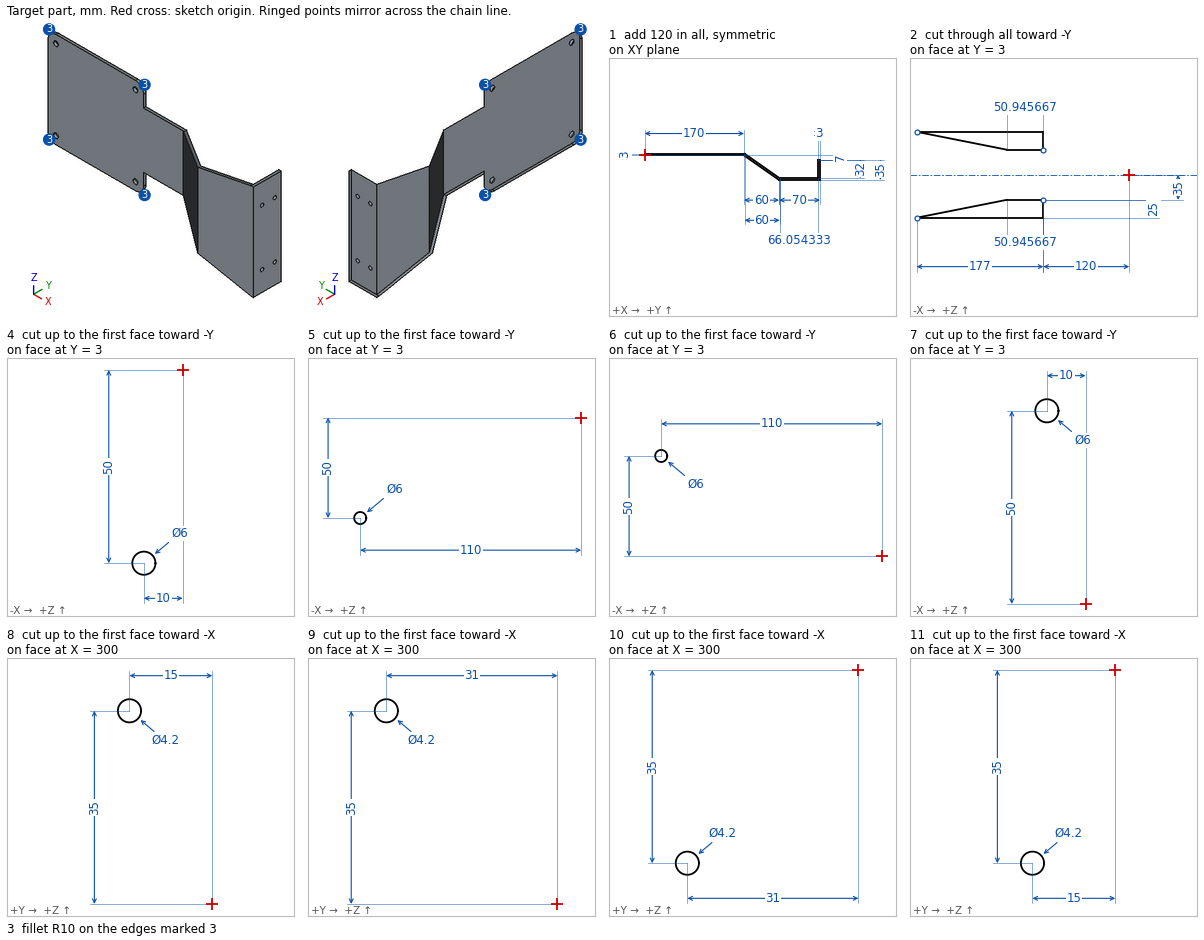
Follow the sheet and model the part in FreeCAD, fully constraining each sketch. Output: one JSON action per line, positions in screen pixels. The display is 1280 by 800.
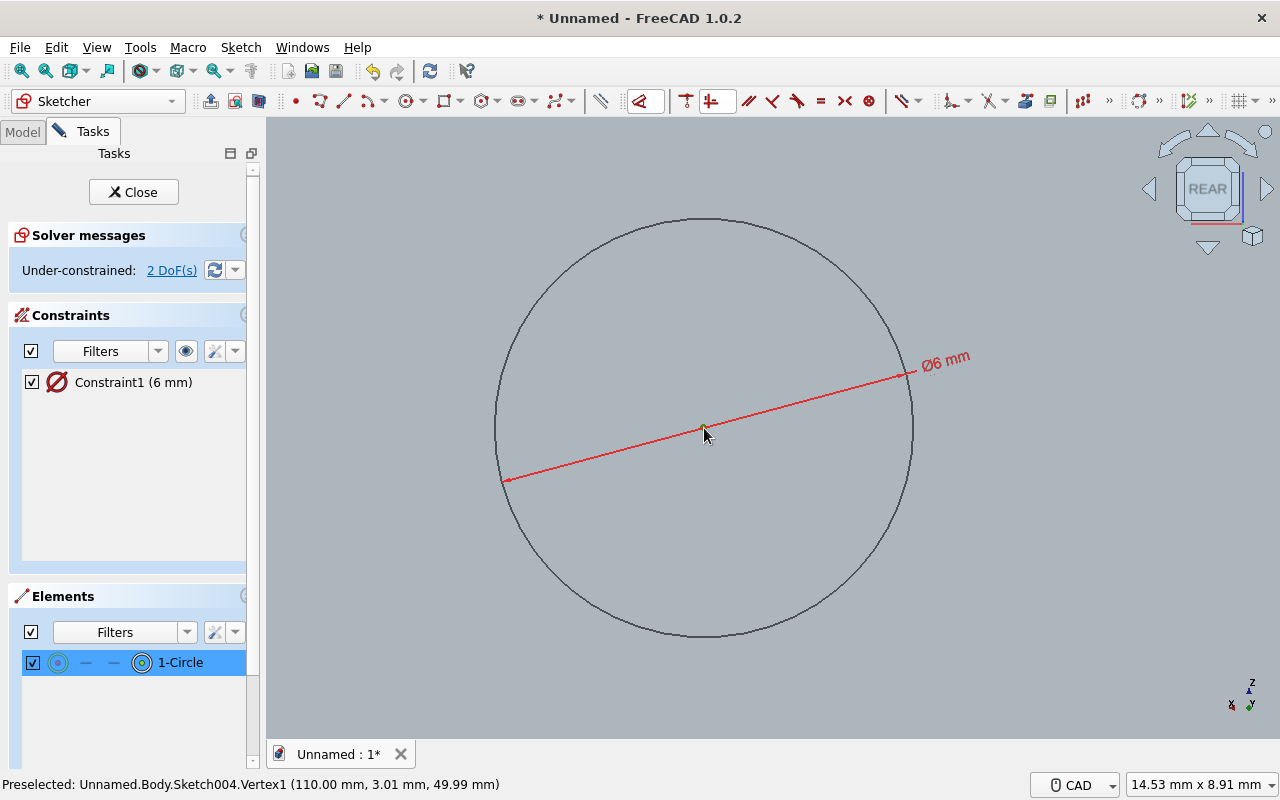
{"action": "left_click", "coordinate": [658, 102]}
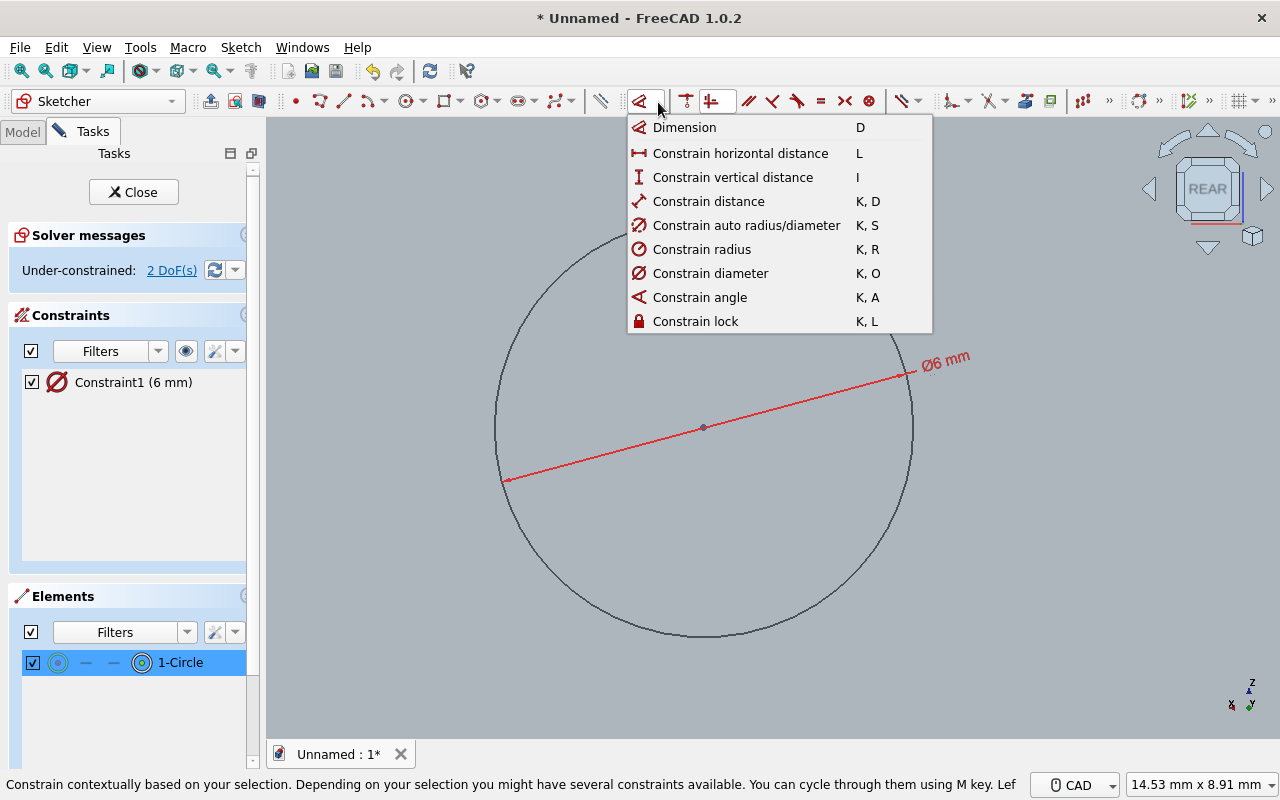
{"action": "left_click", "coordinate": [780, 177]}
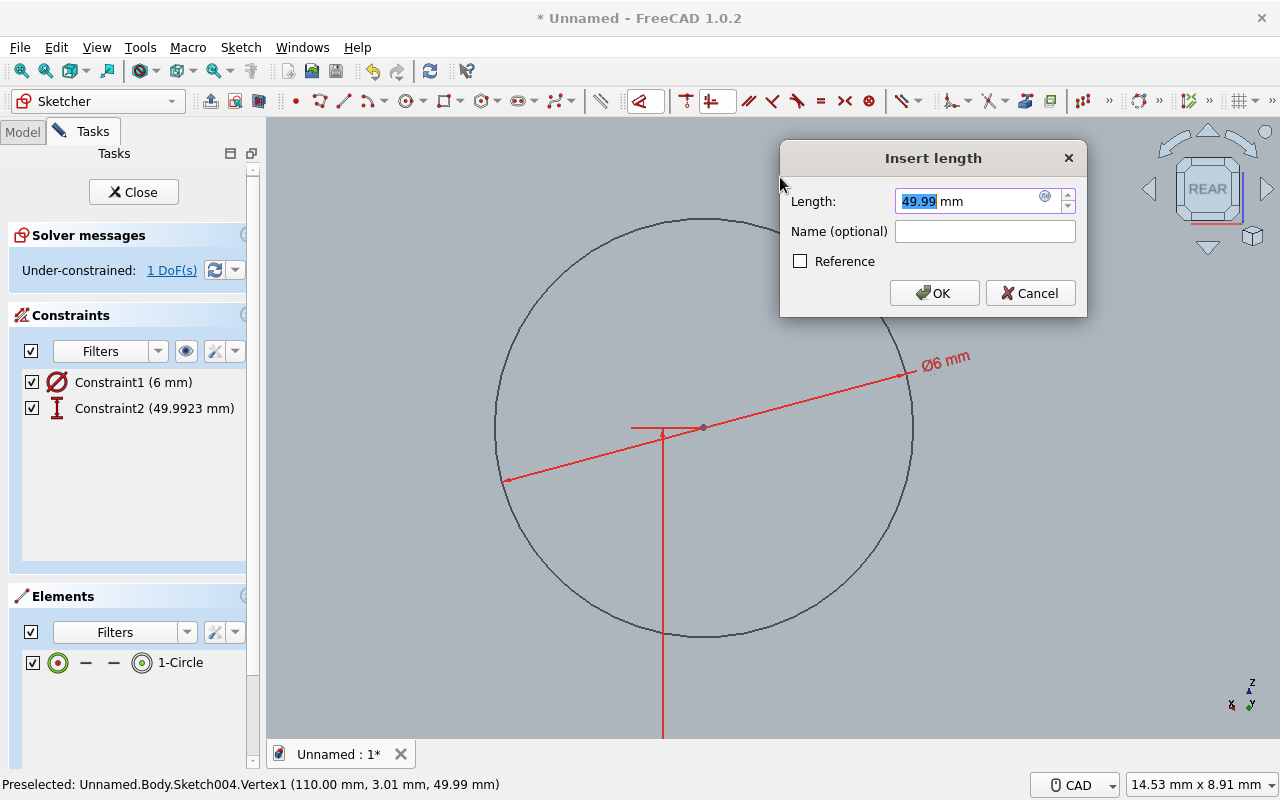
{"action": "type", "text": "50"}
{"action": "key", "text": "Return"}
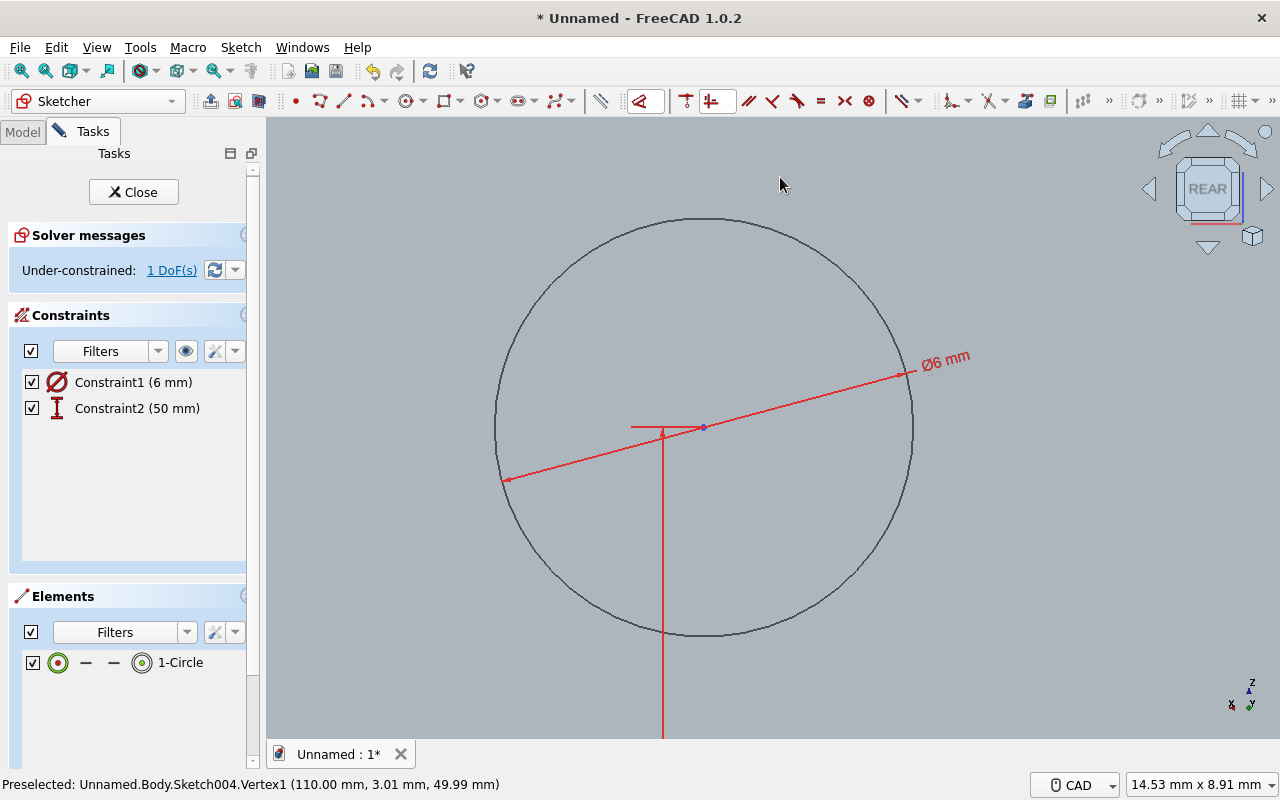
{"action": "left_click", "coordinate": [704, 427]}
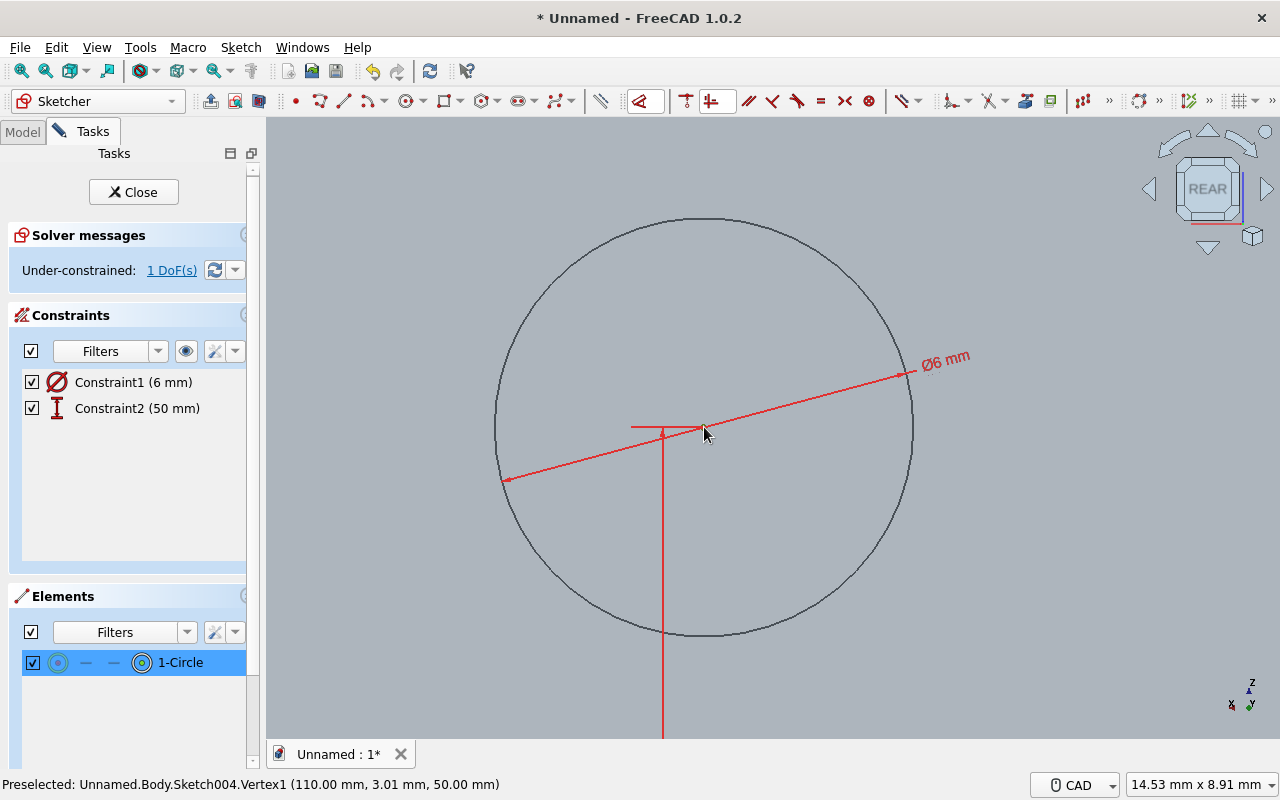
{"action": "left_click", "coordinate": [658, 102]}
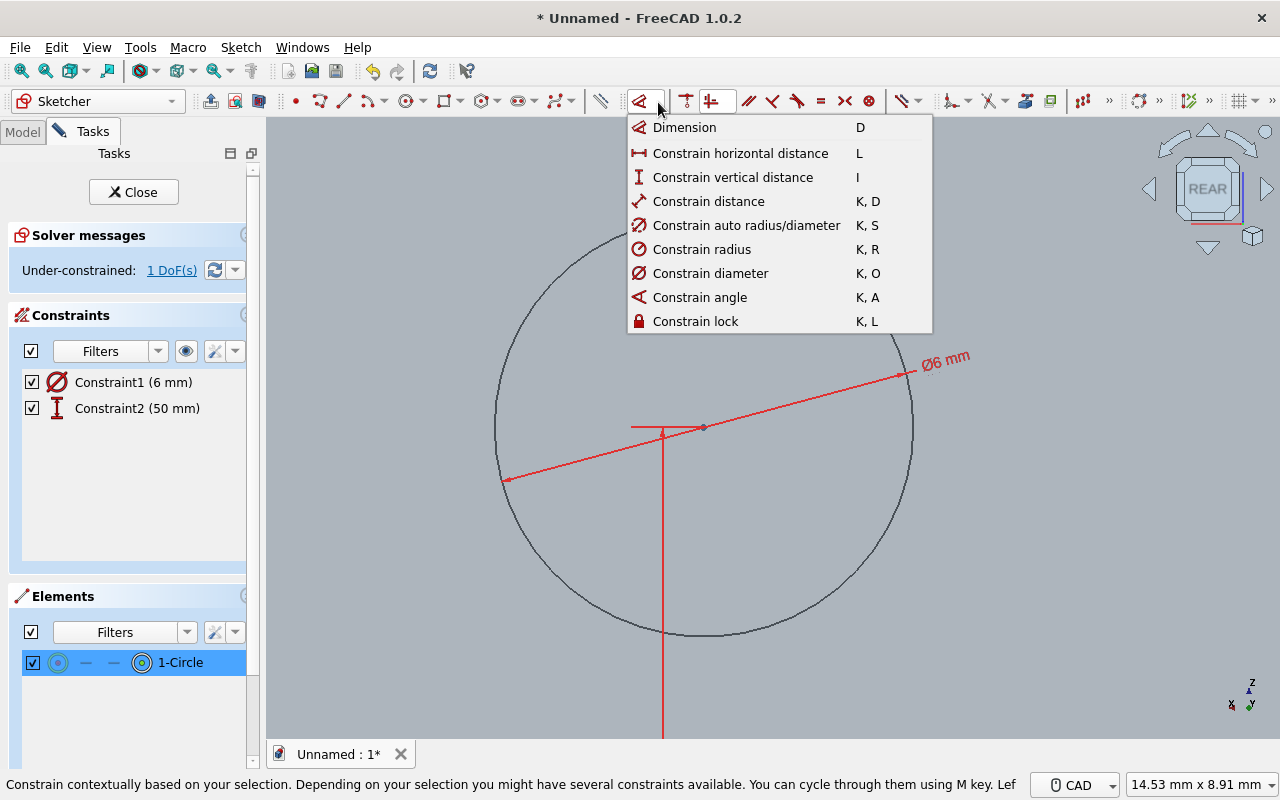
{"action": "left_click", "coordinate": [780, 153]}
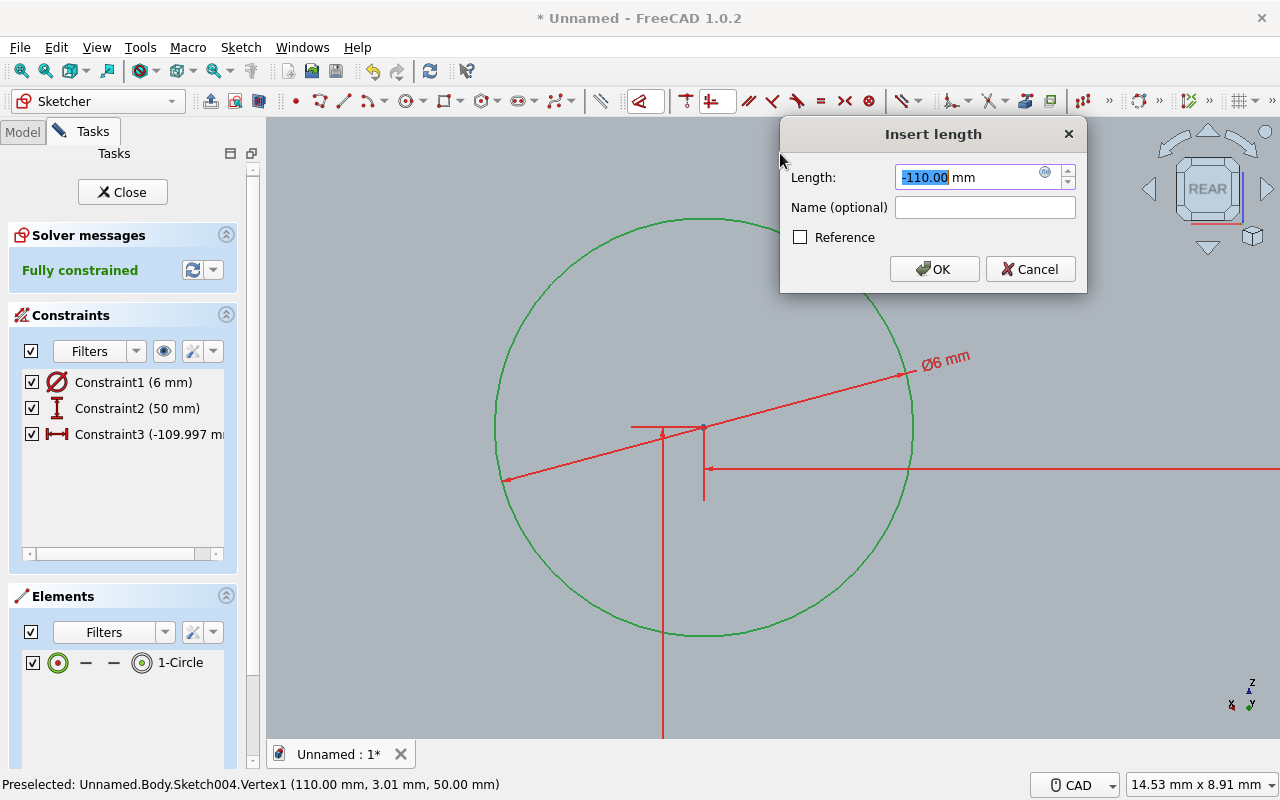
{"action": "type", "text": "-110"}
{"action": "key", "text": "Return"}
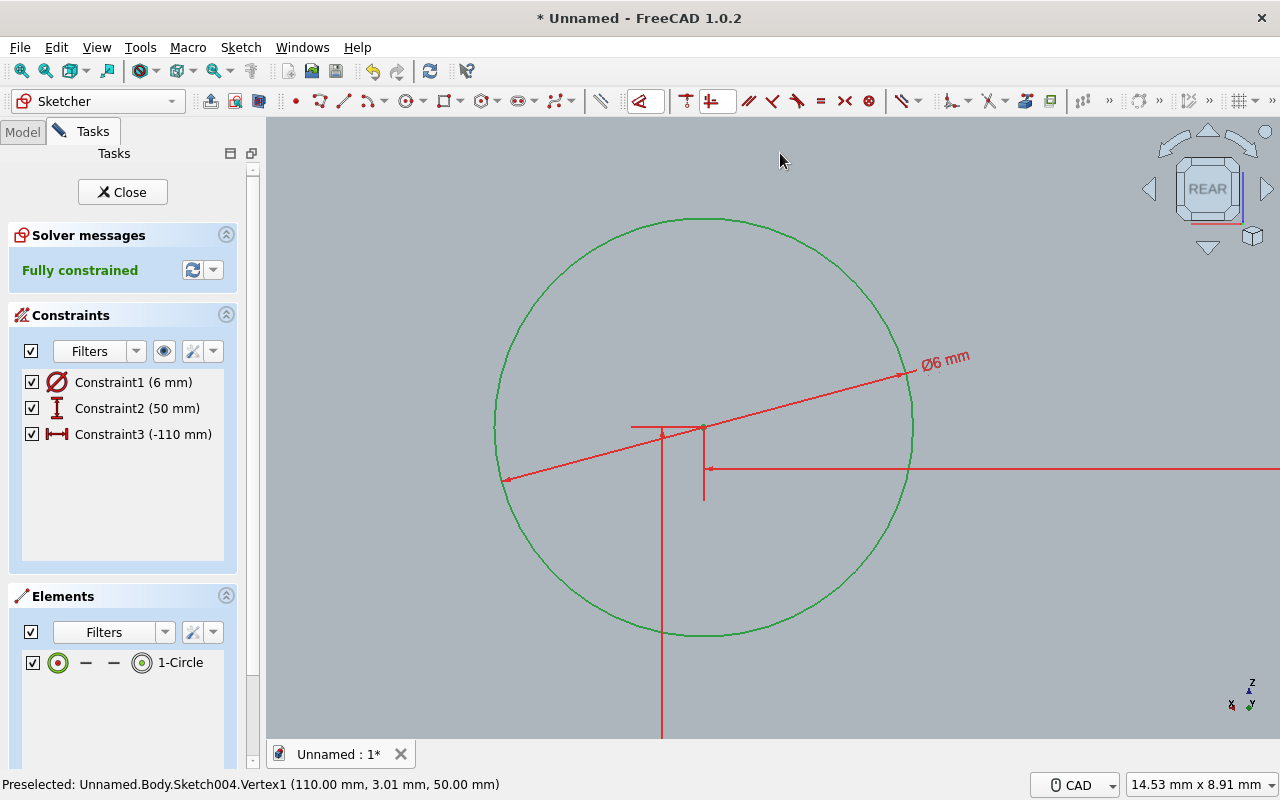
{"action": "left_click", "coordinate": [123, 192]}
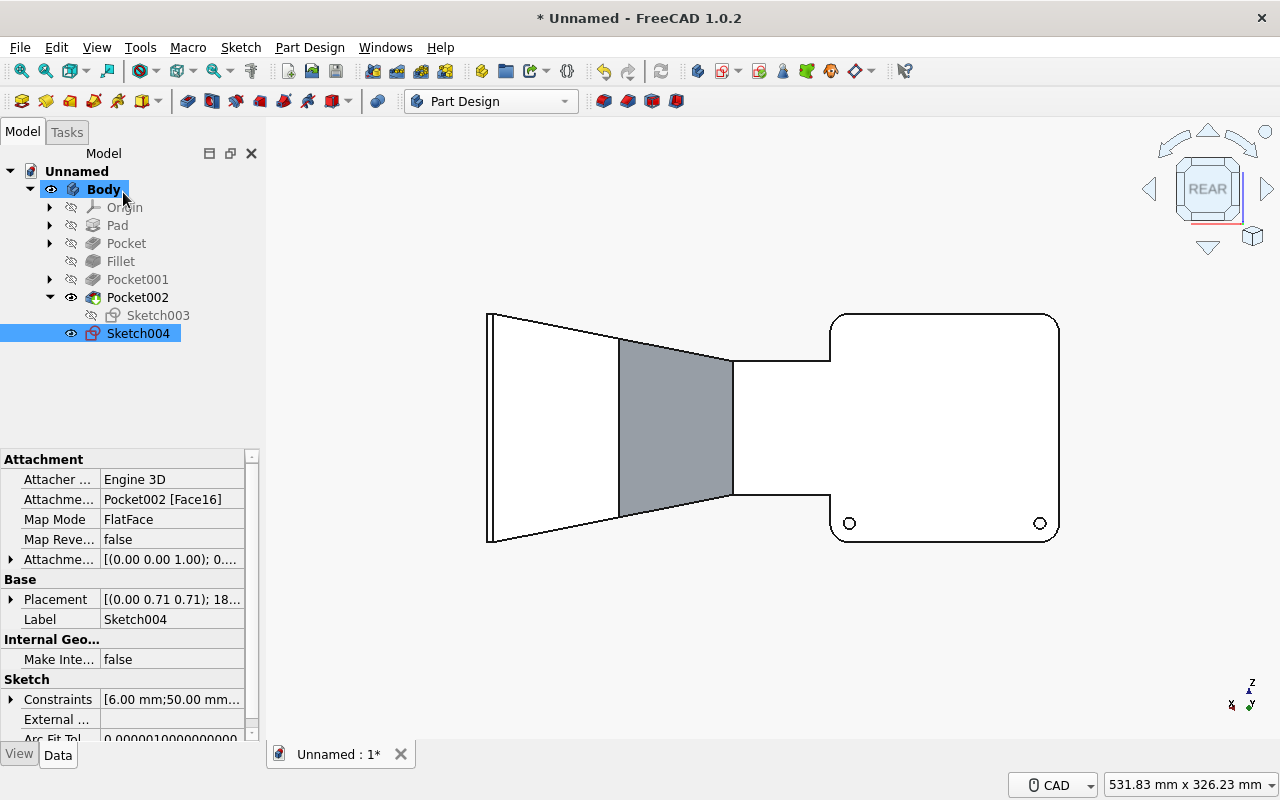
{"action": "left_click", "coordinate": [188, 102]}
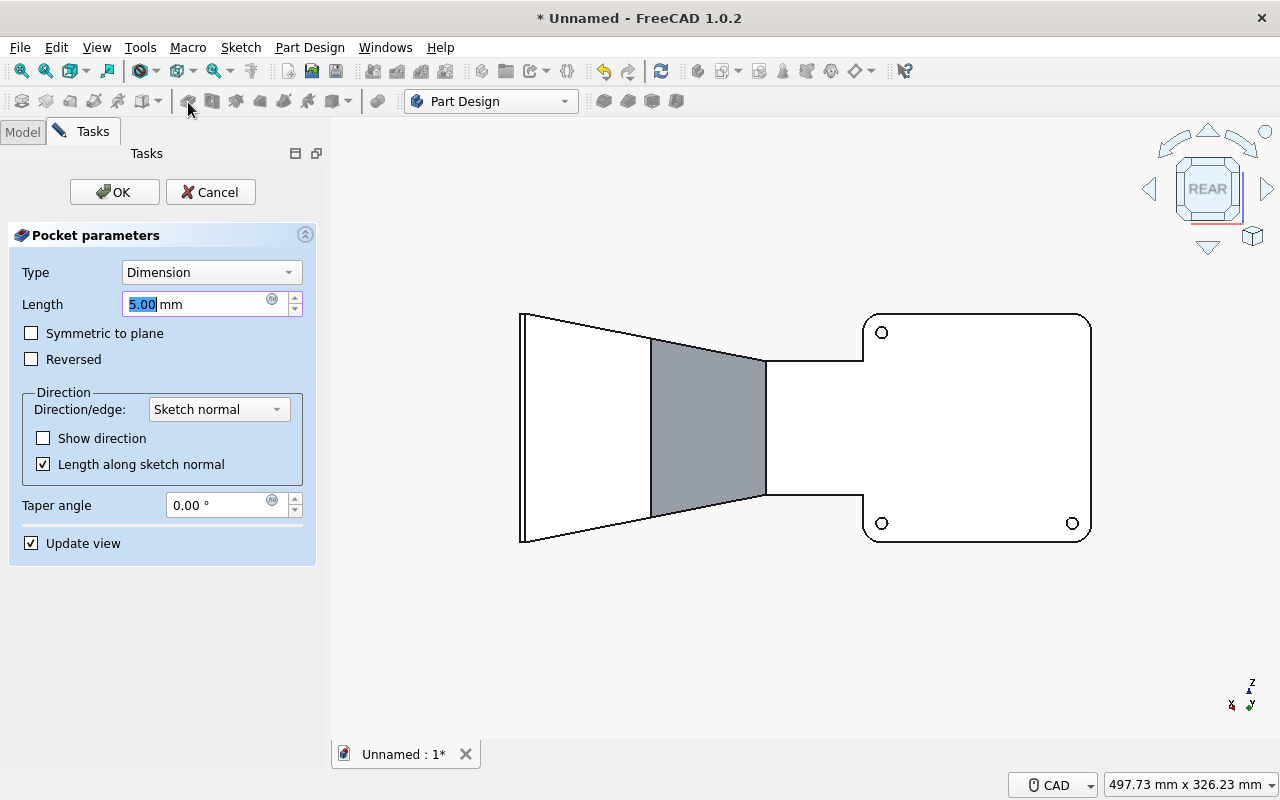
{"action": "left_click", "coordinate": [212, 272]}